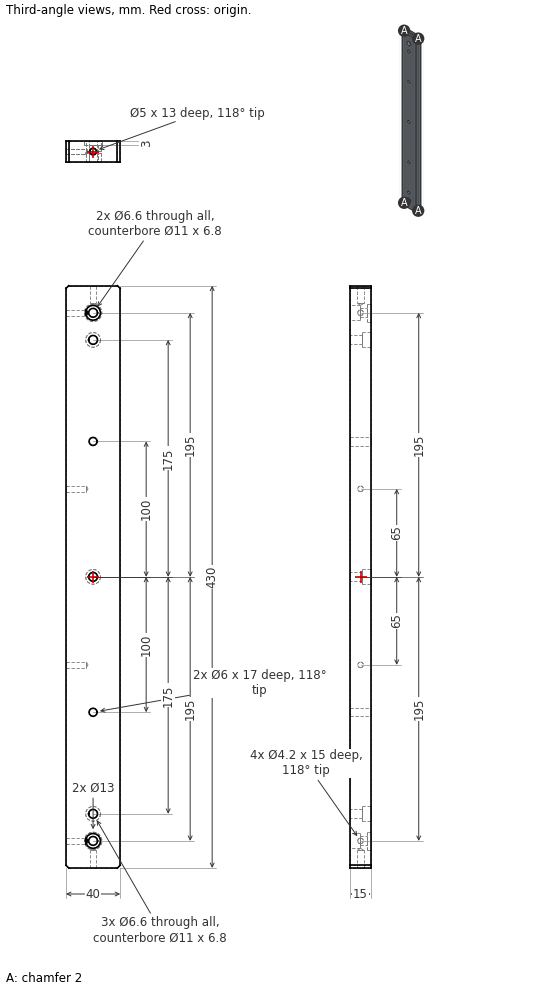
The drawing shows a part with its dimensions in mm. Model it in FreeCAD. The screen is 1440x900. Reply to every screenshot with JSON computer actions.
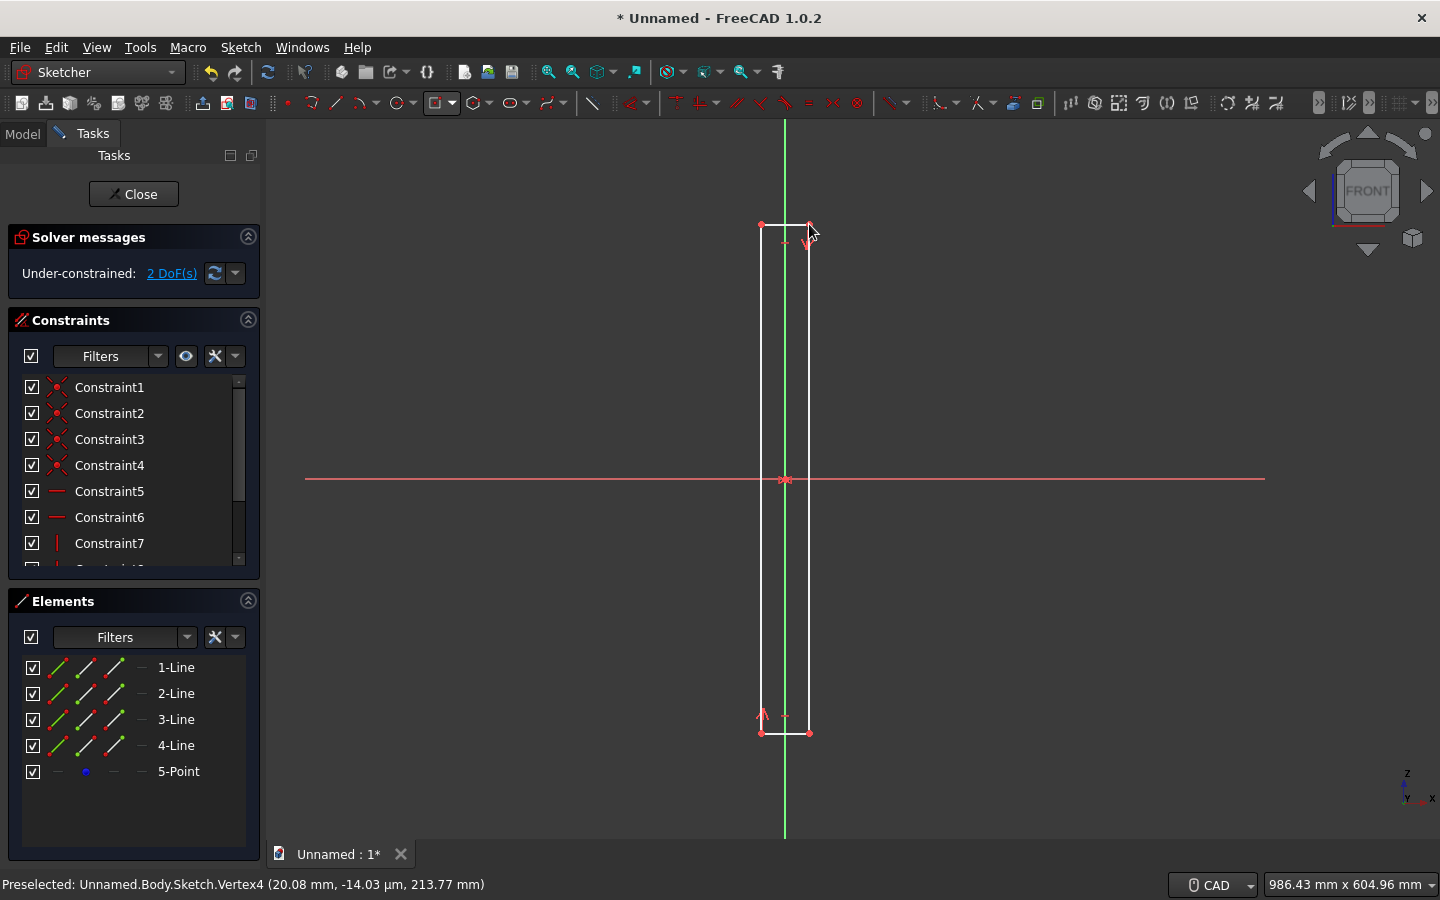
{"action": "left_click", "coordinate": [630, 104]}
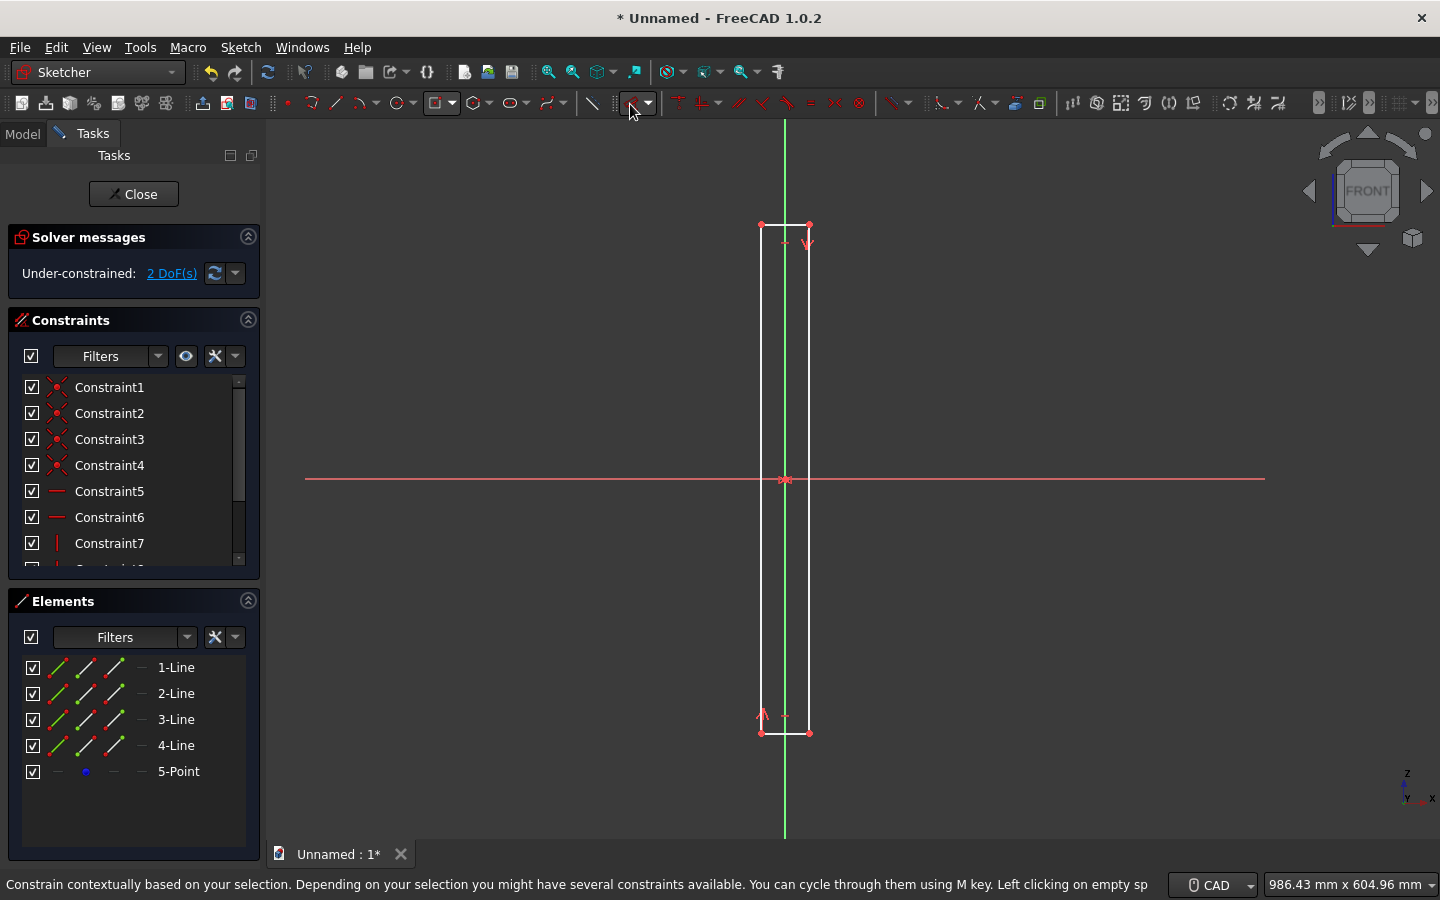
{"action": "scroll", "coordinate": [776, 734], "scroll_direction": "up", "scroll_amount": 2}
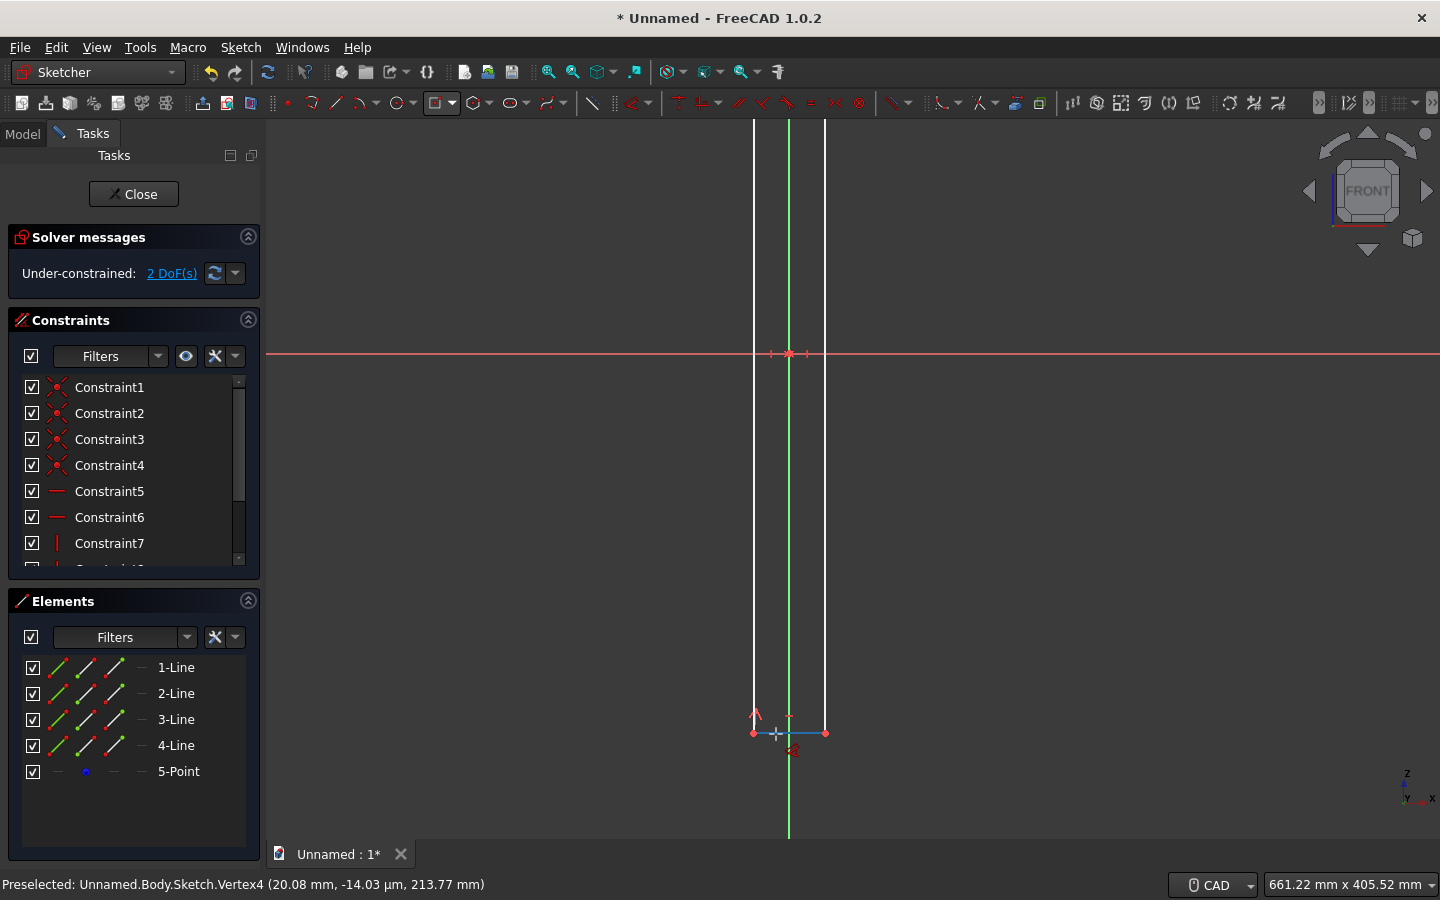
{"action": "left_click", "coordinate": [775, 733]}
{"action": "left_click", "coordinate": [773, 767]}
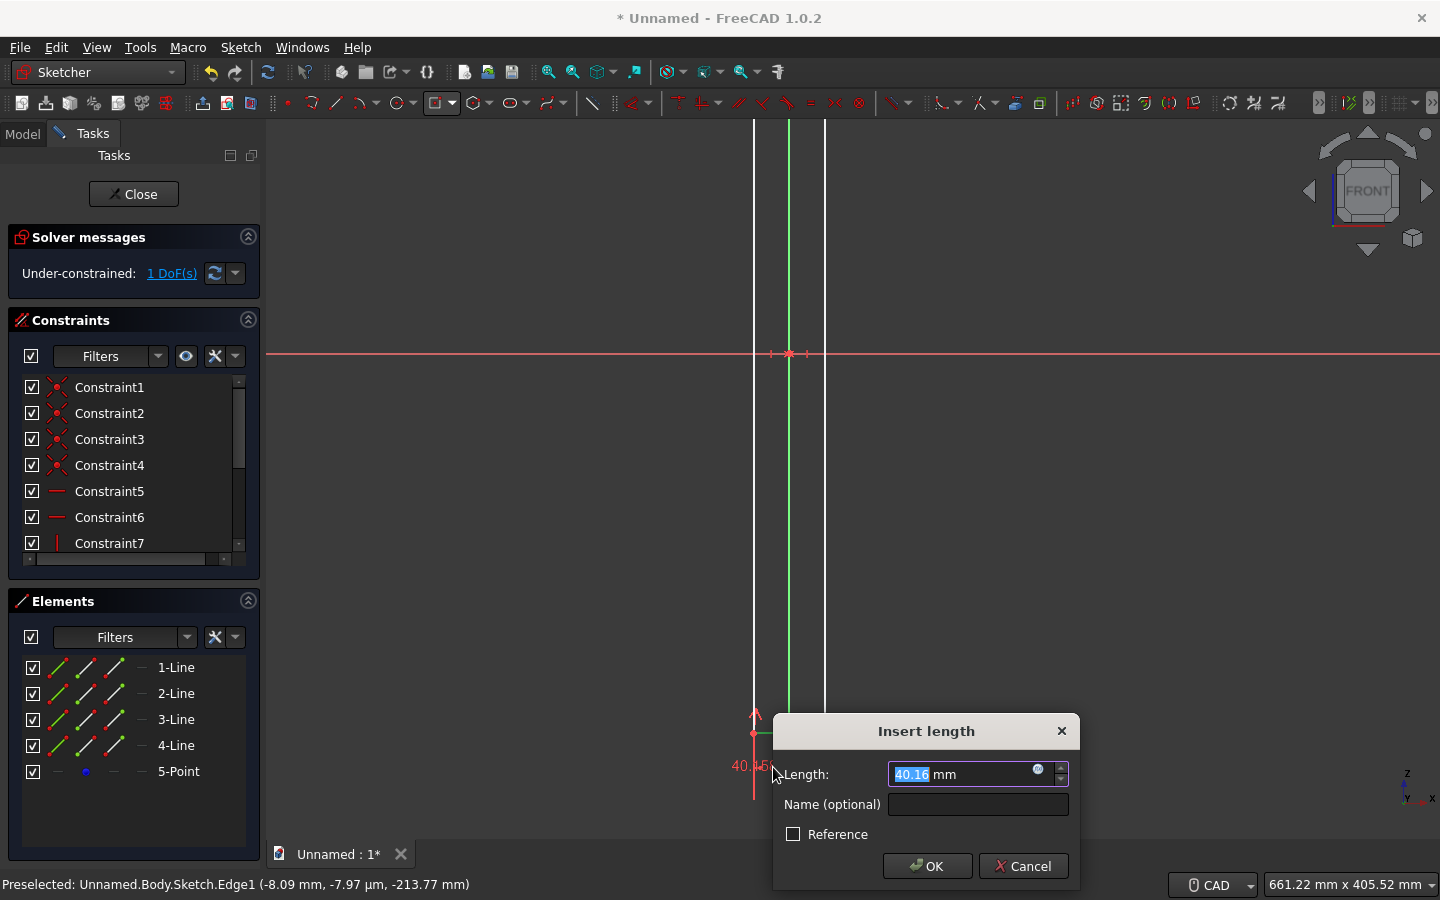
{"action": "type", "text": "40"}
{"action": "key", "text": "Return"}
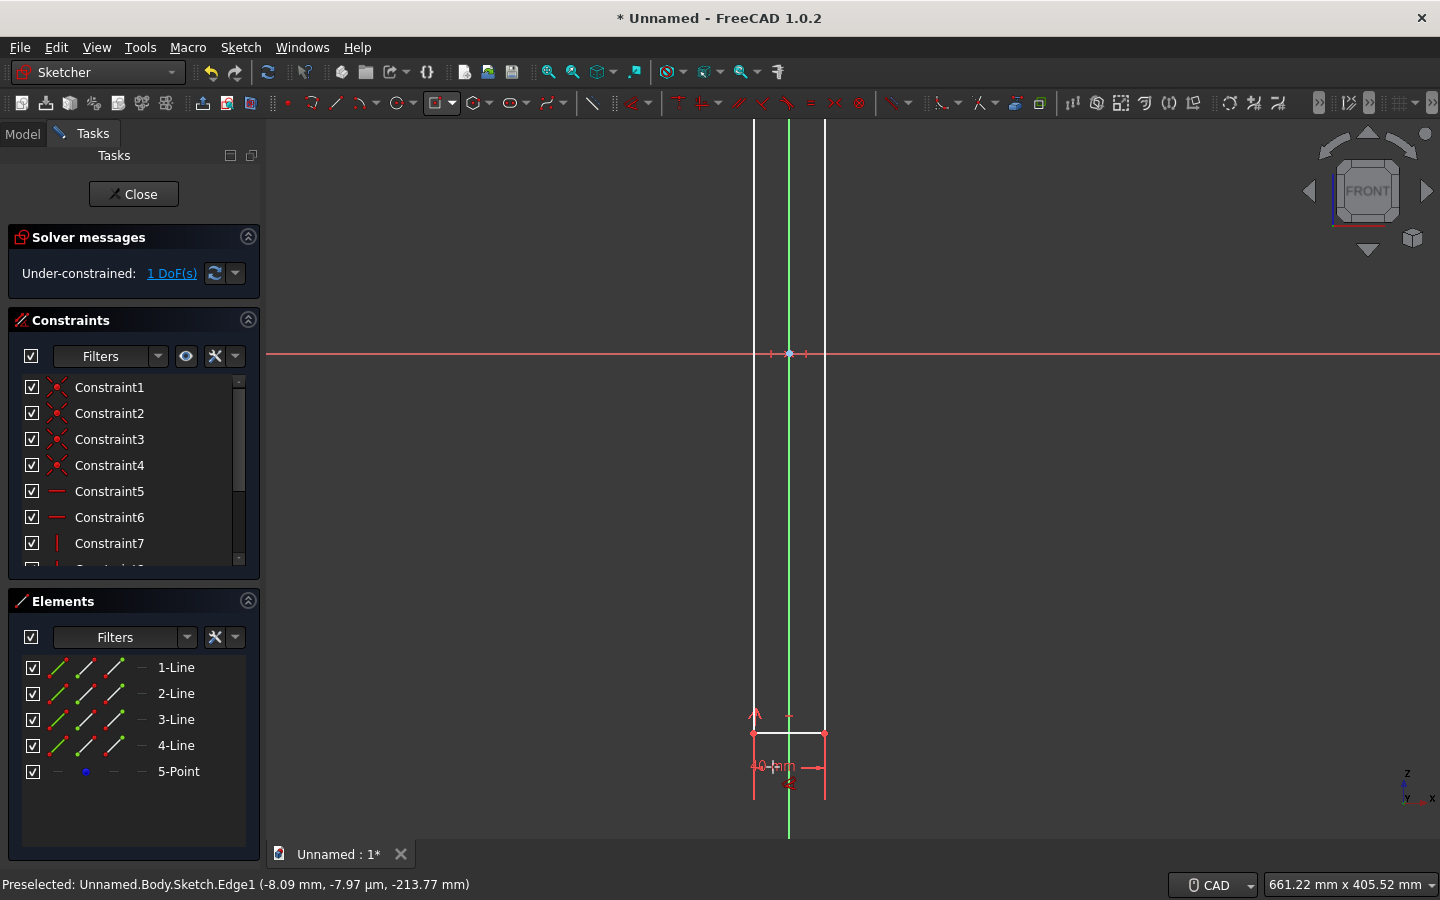
{"action": "left_click", "coordinate": [825, 506]}
{"action": "left_click", "coordinate": [859, 440]}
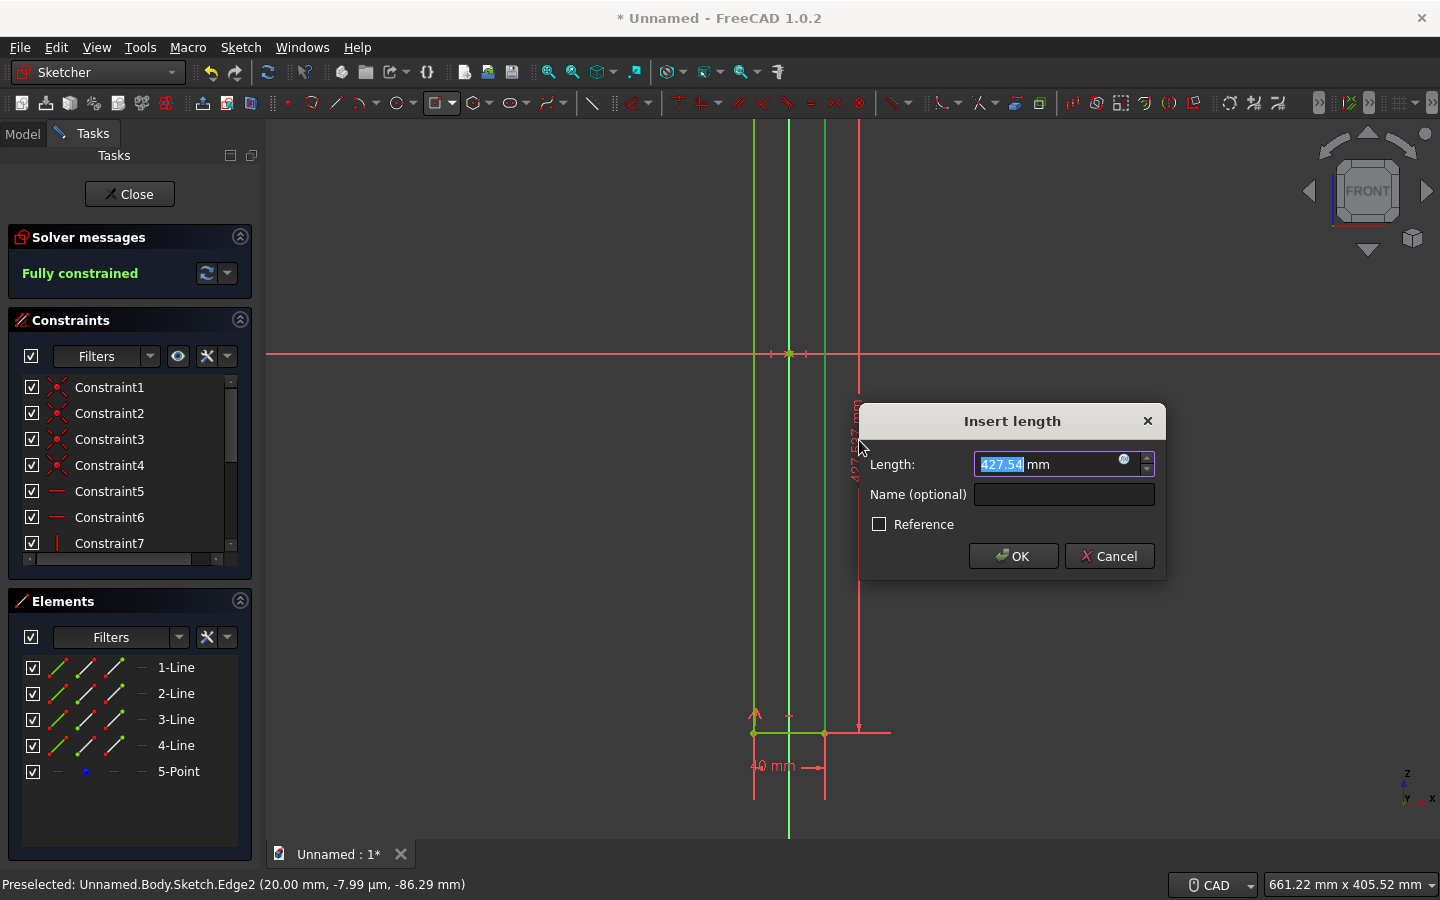
{"action": "type", "text": "430"}
{"action": "key", "text": "Return"}
{"action": "key", "text": "Escape"}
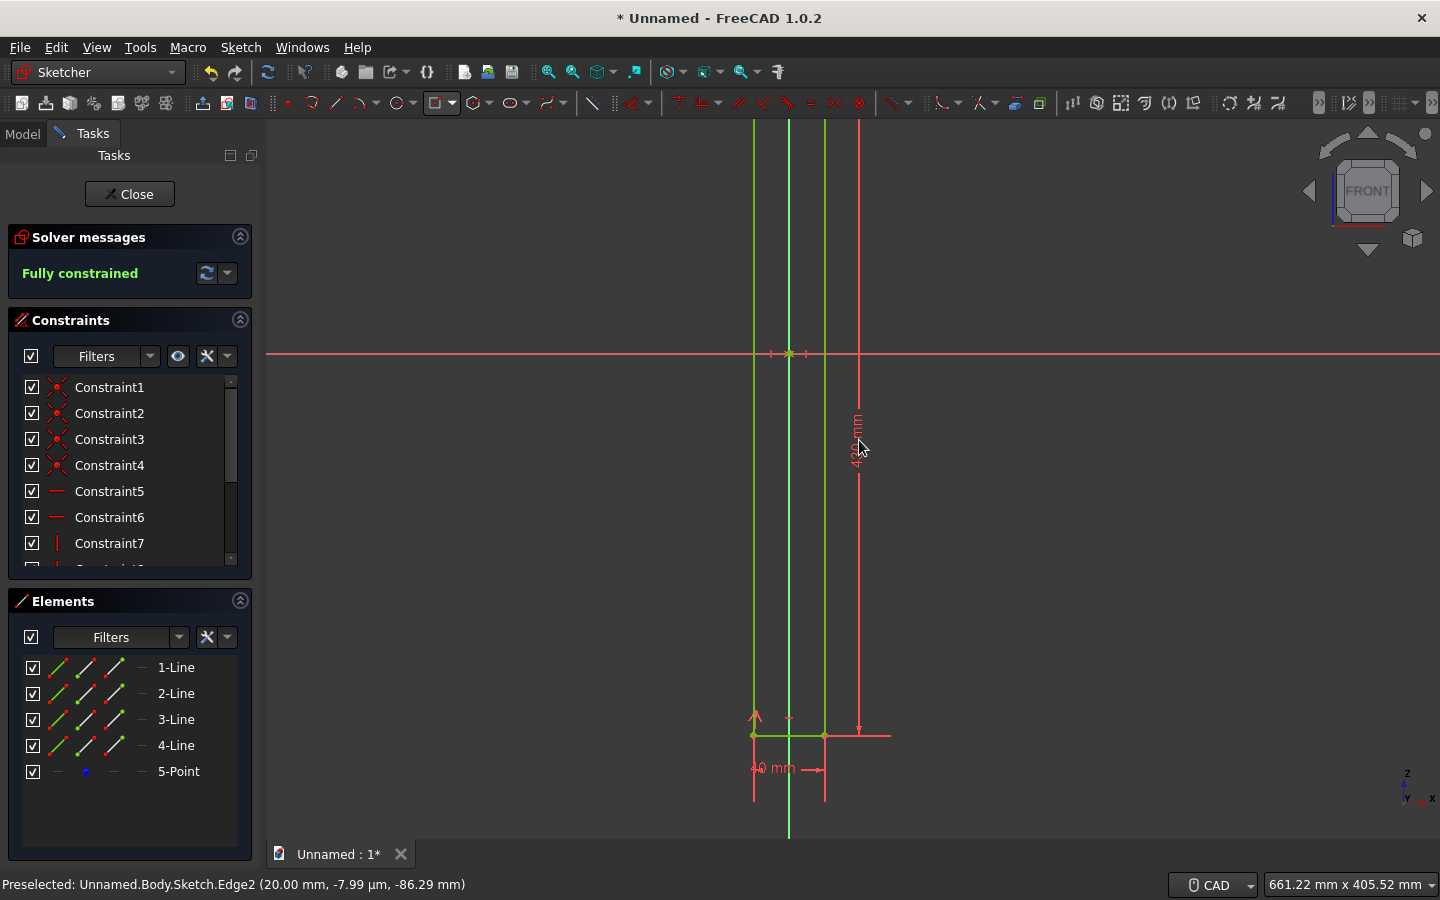
{"action": "left_click", "coordinate": [130, 194]}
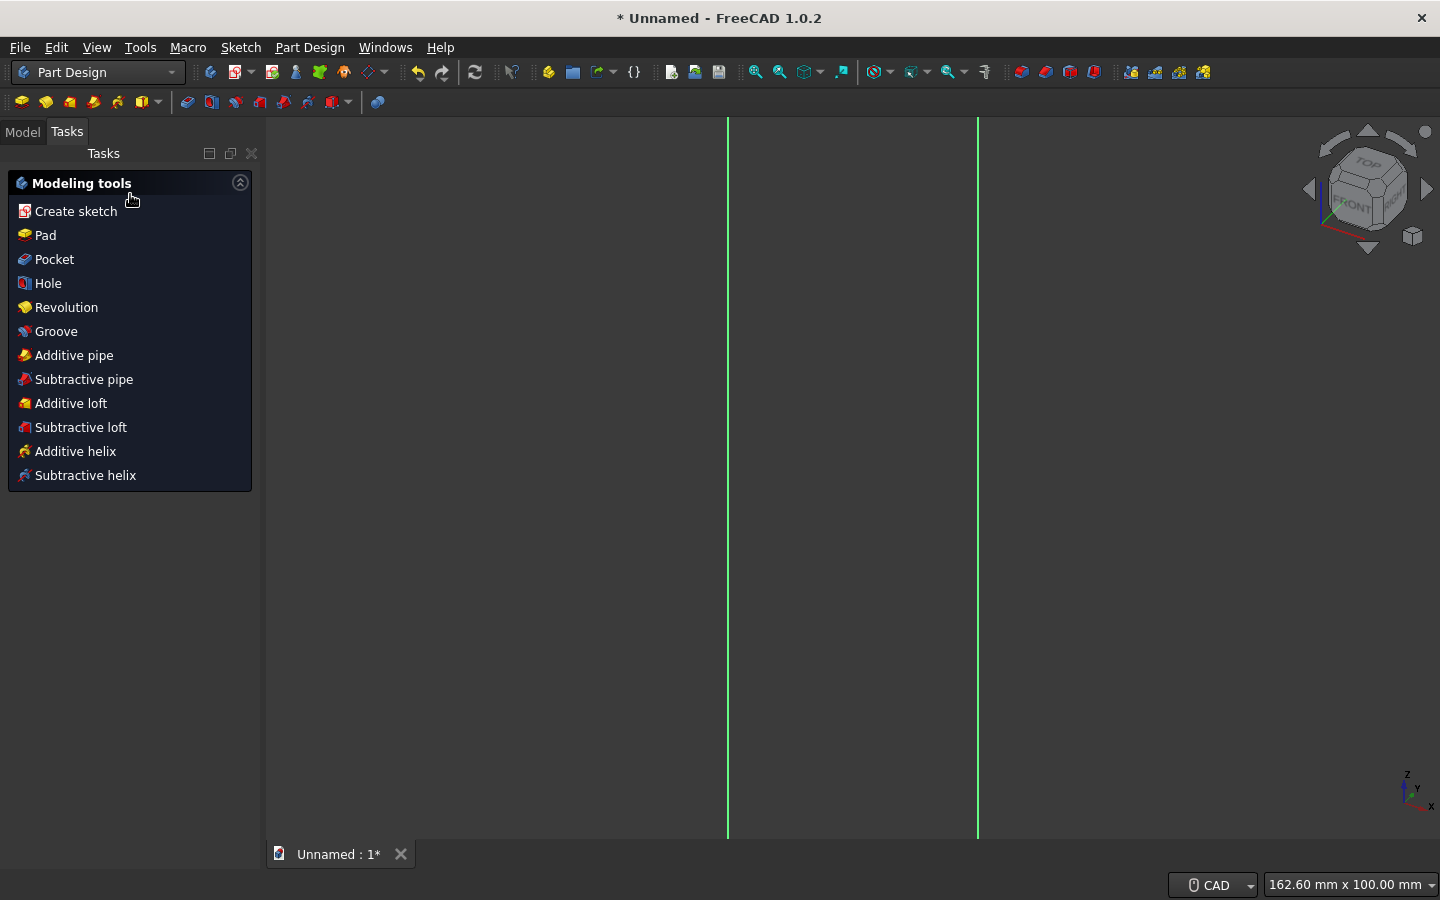
{"action": "left_click", "coordinate": [22, 102]}